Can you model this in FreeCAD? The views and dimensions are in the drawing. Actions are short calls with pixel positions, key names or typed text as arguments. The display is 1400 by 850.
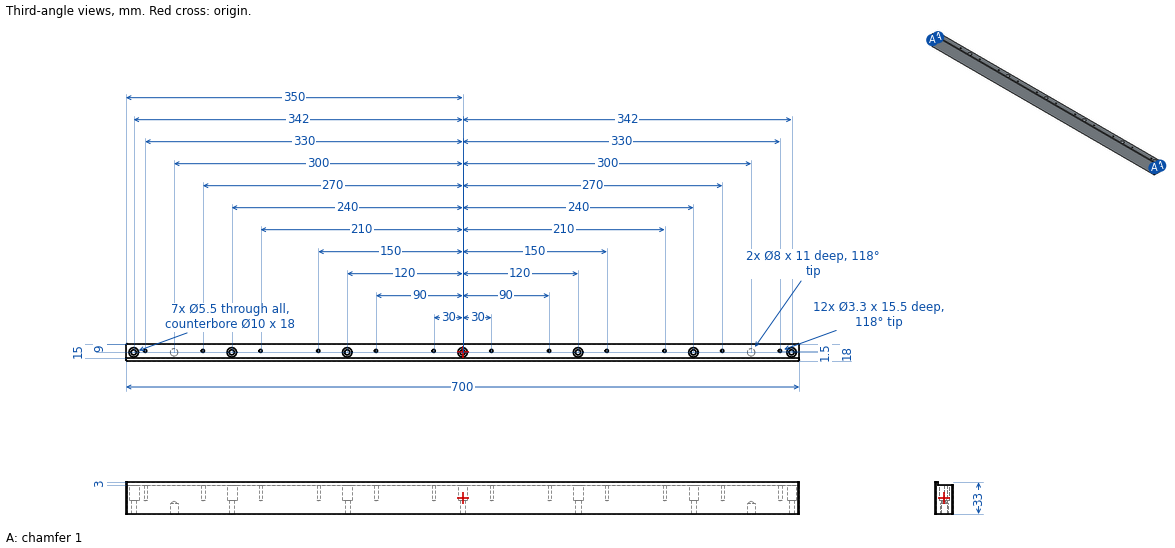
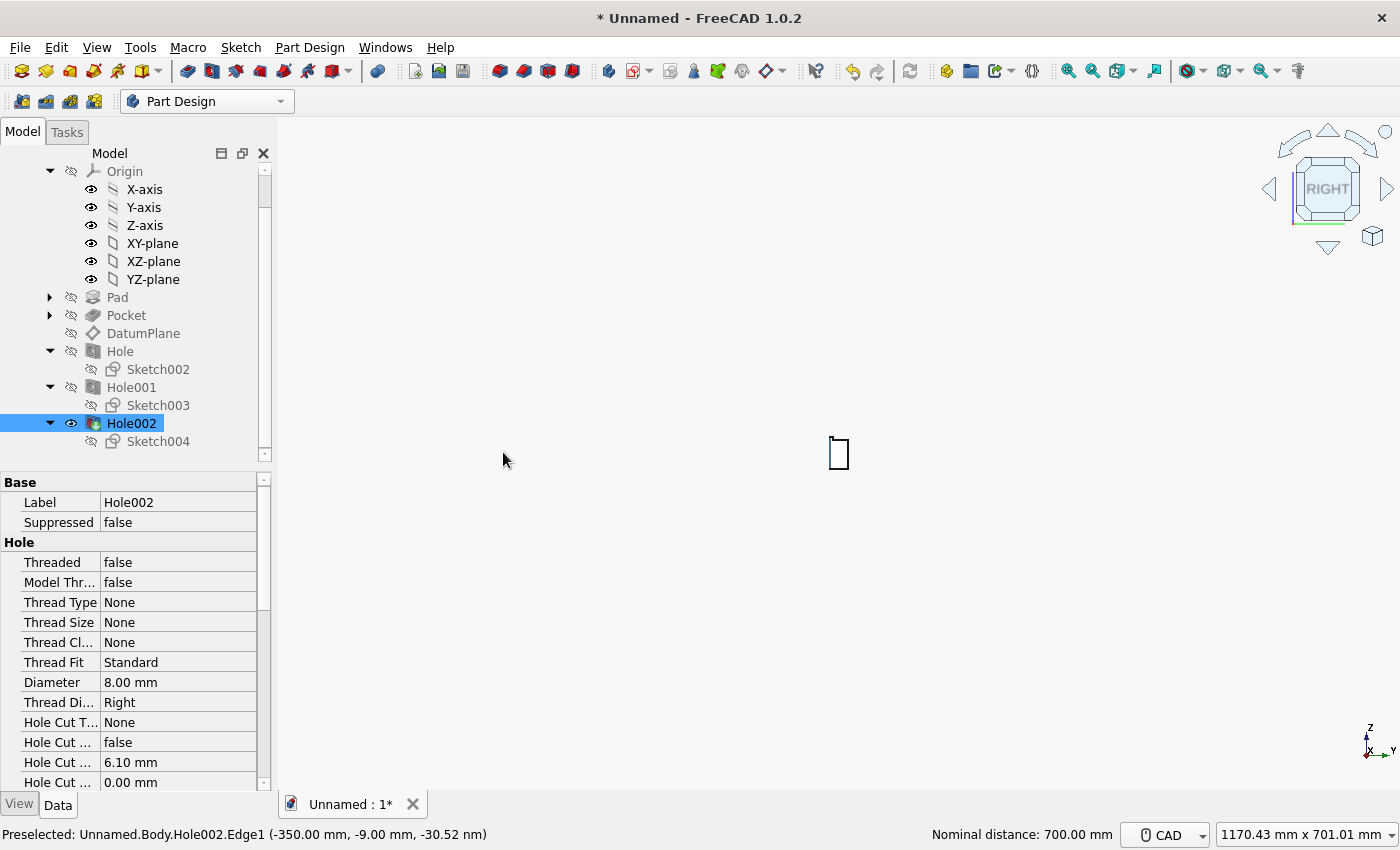
key(v)
key(f)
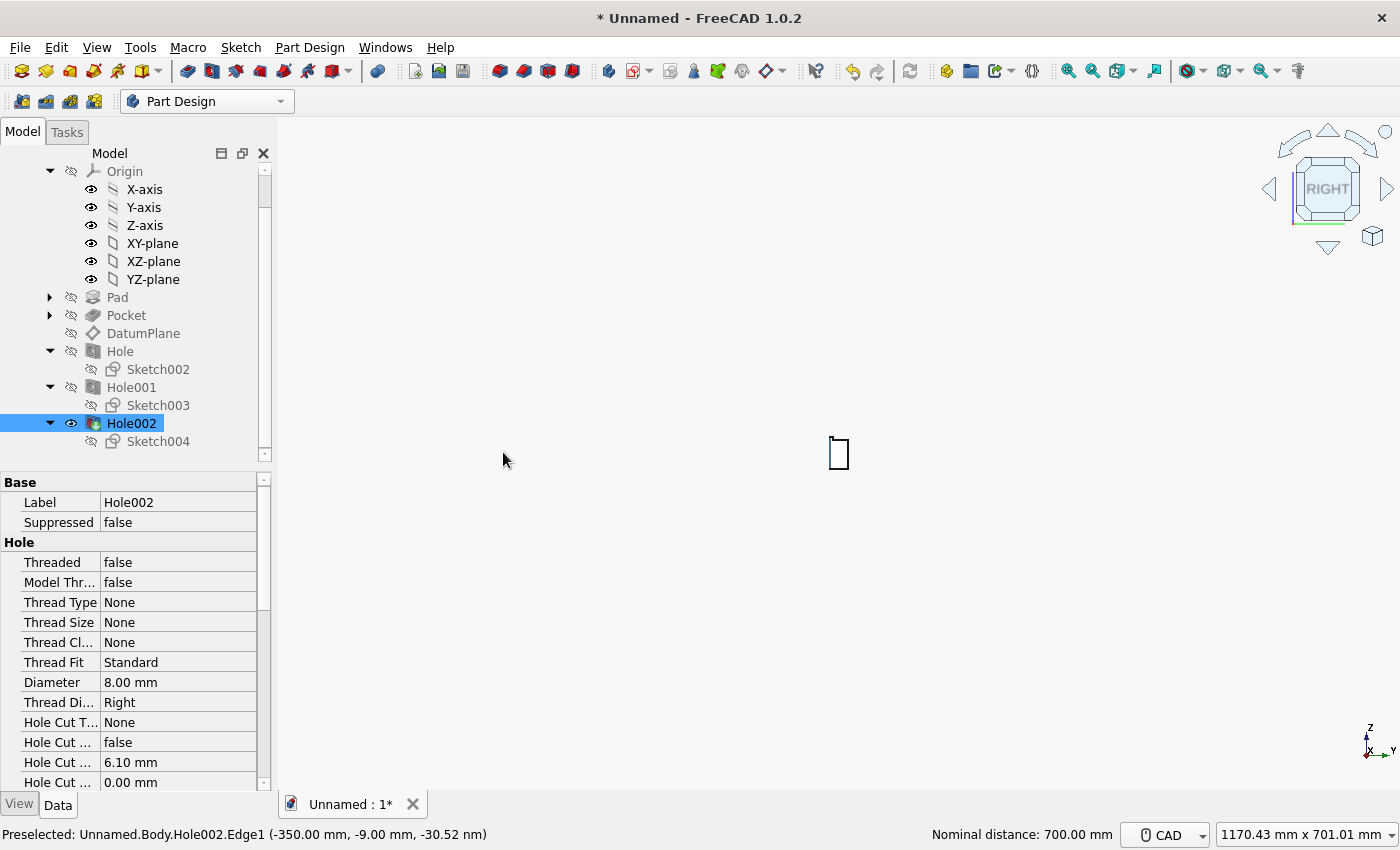
click(848, 453, ctrl)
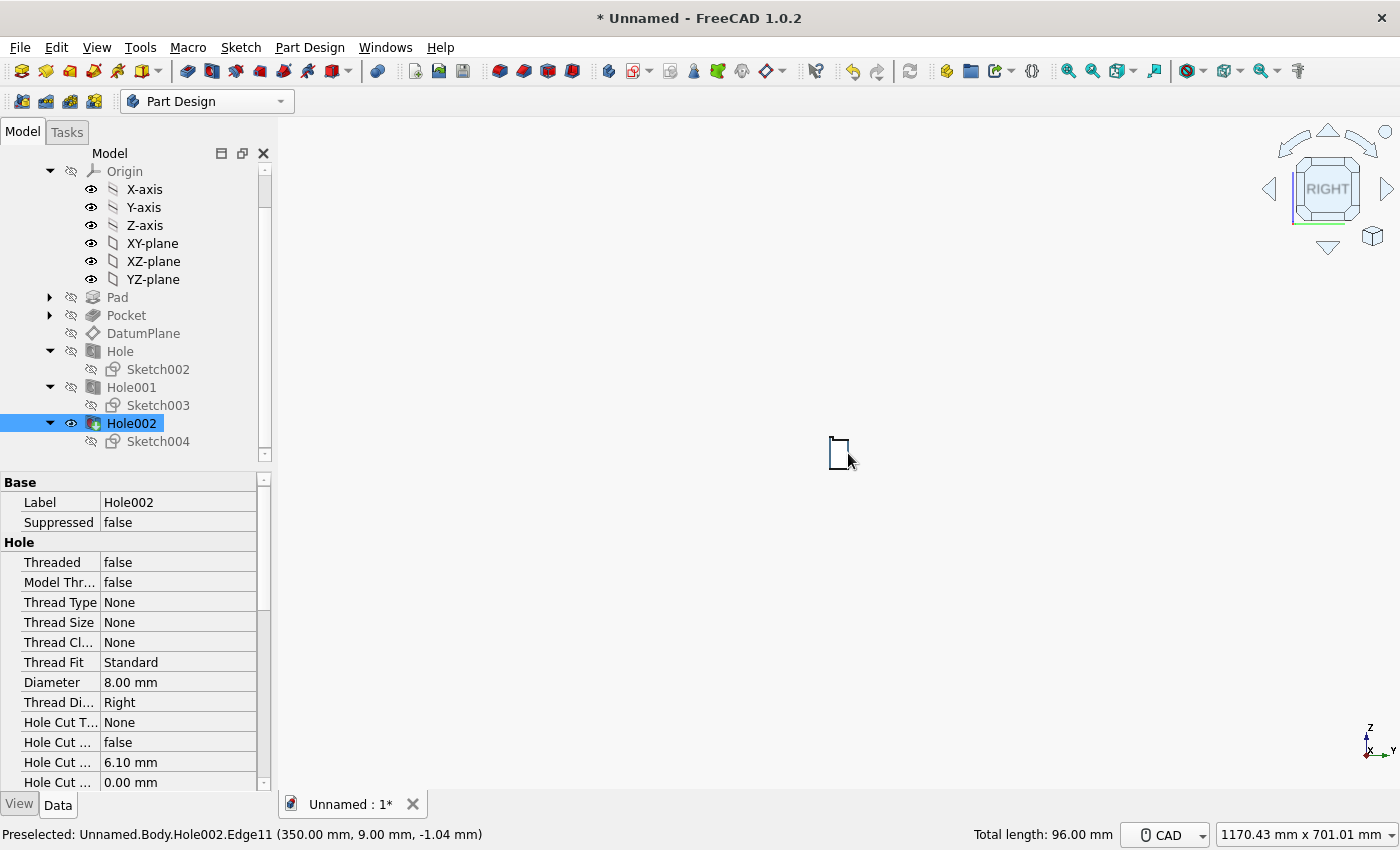
key(5)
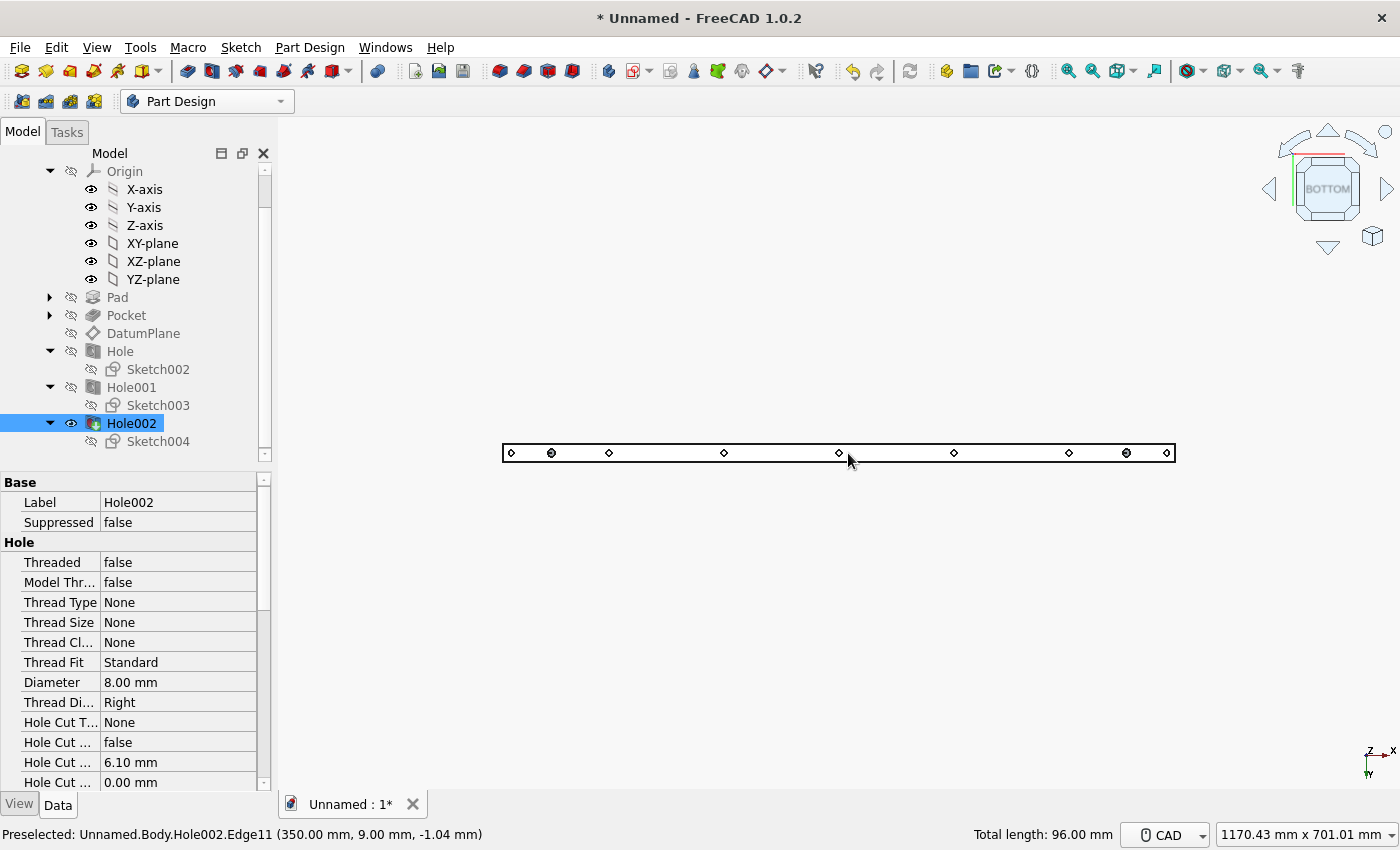
key(4)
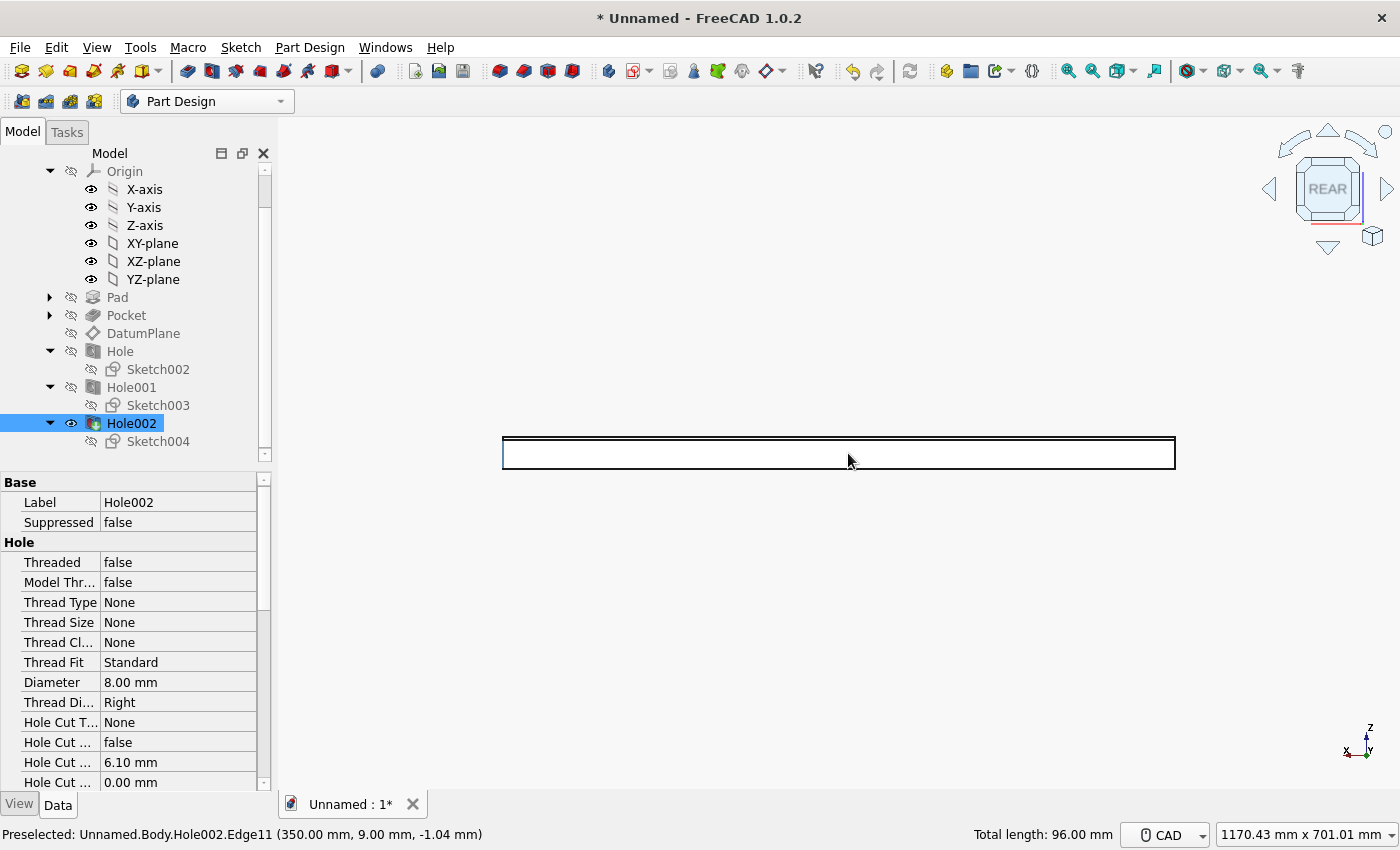
click(1175, 453, ctrl)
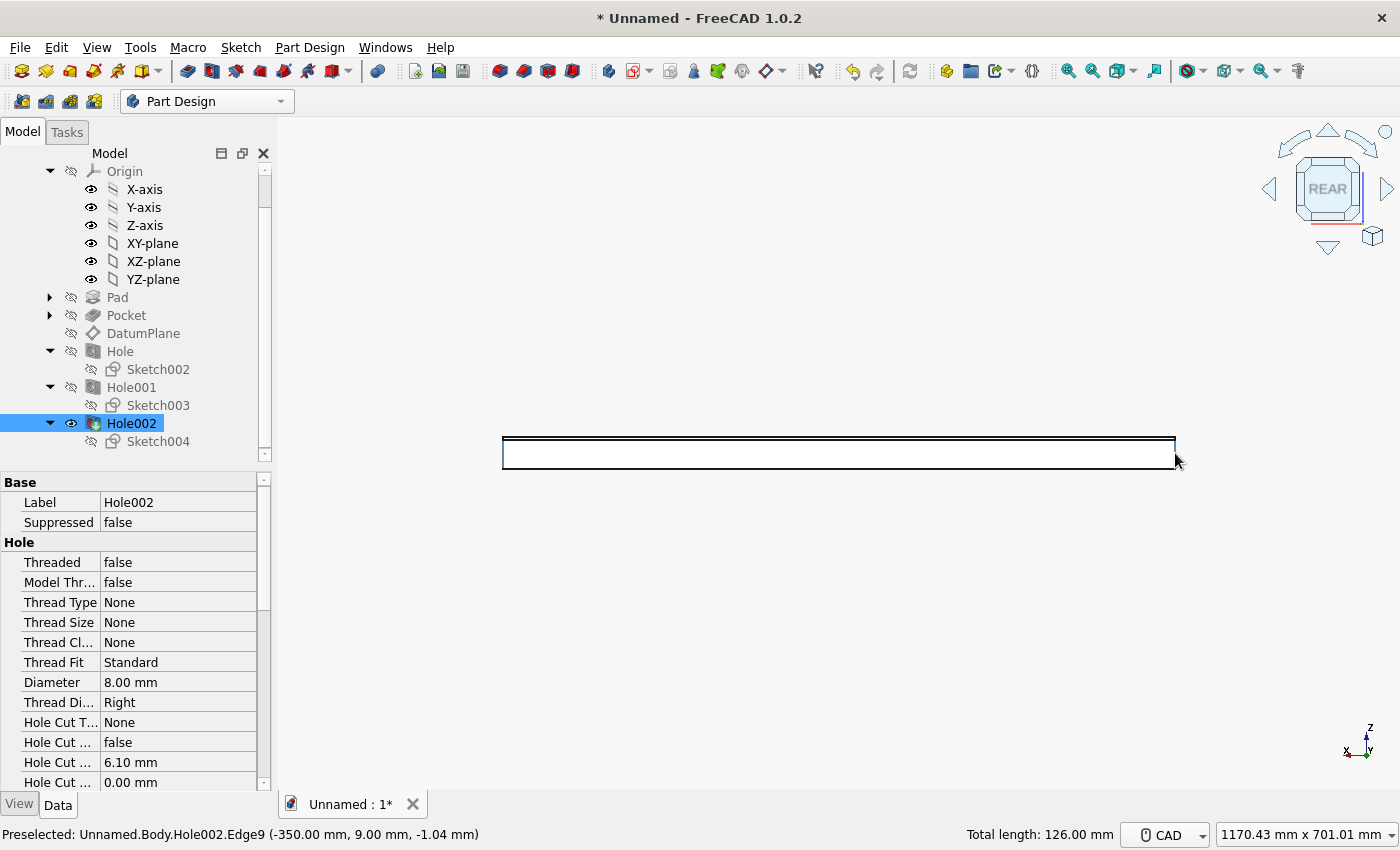
click(524, 72)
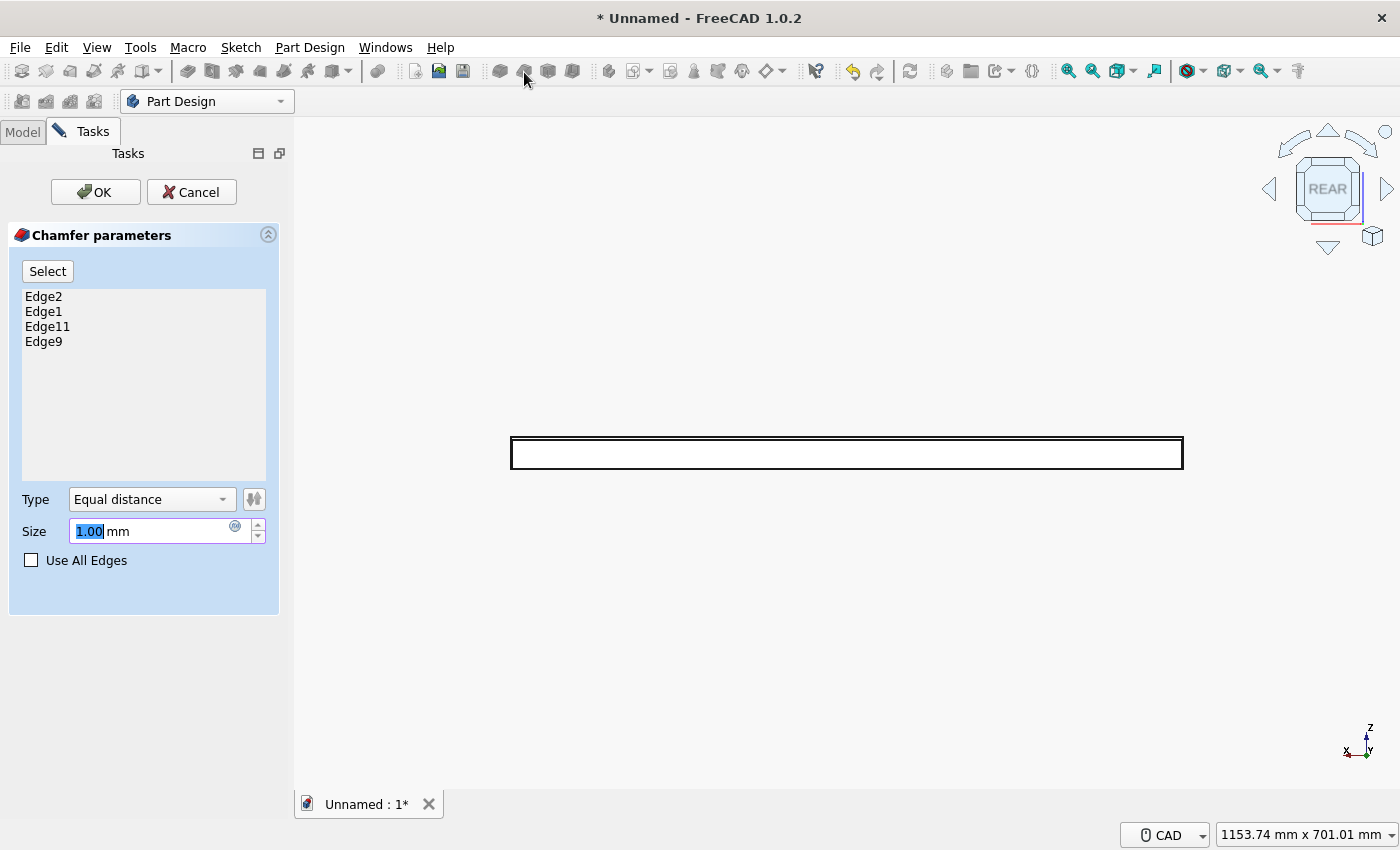
text(1)
key(Tab)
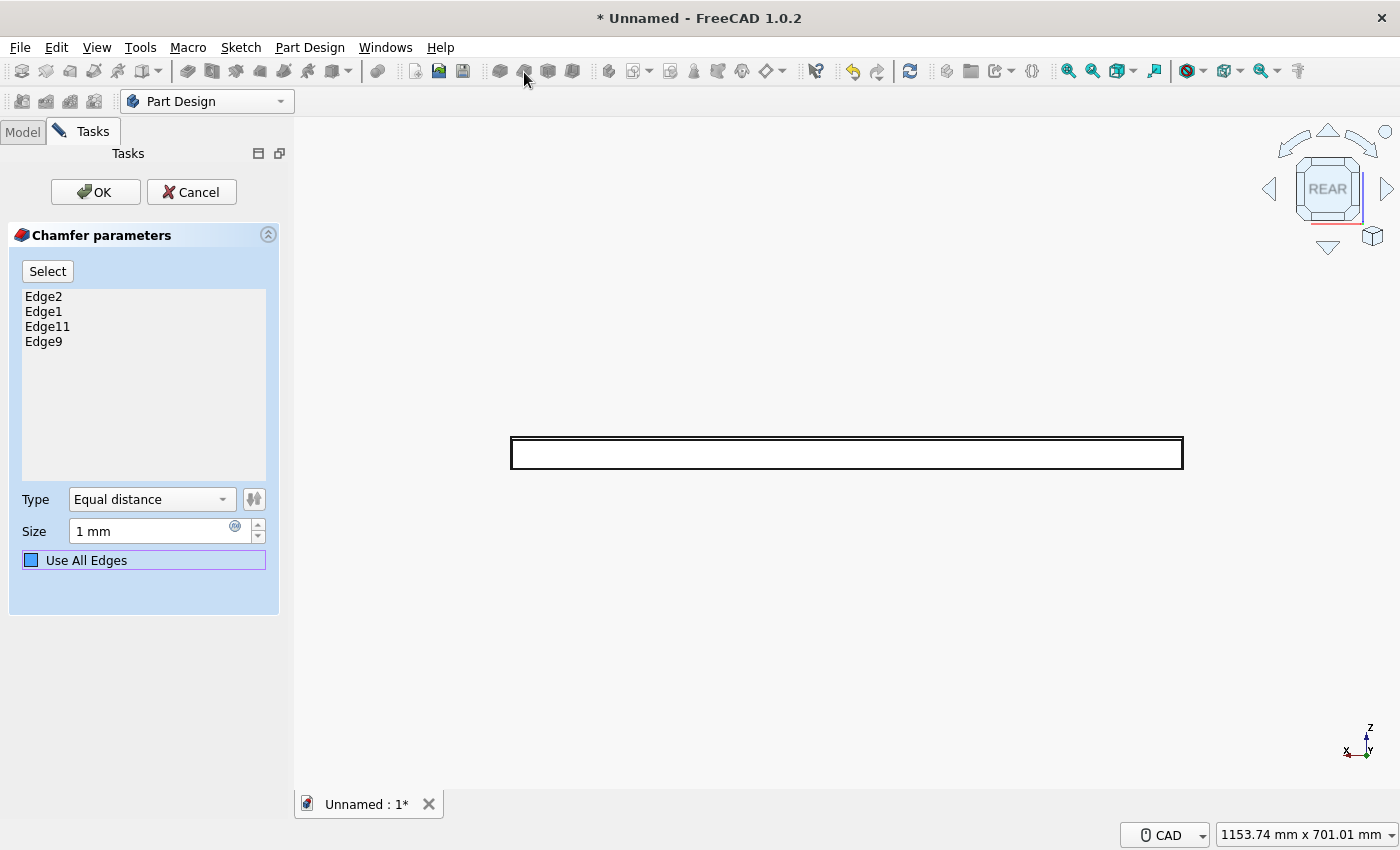
click(96, 192)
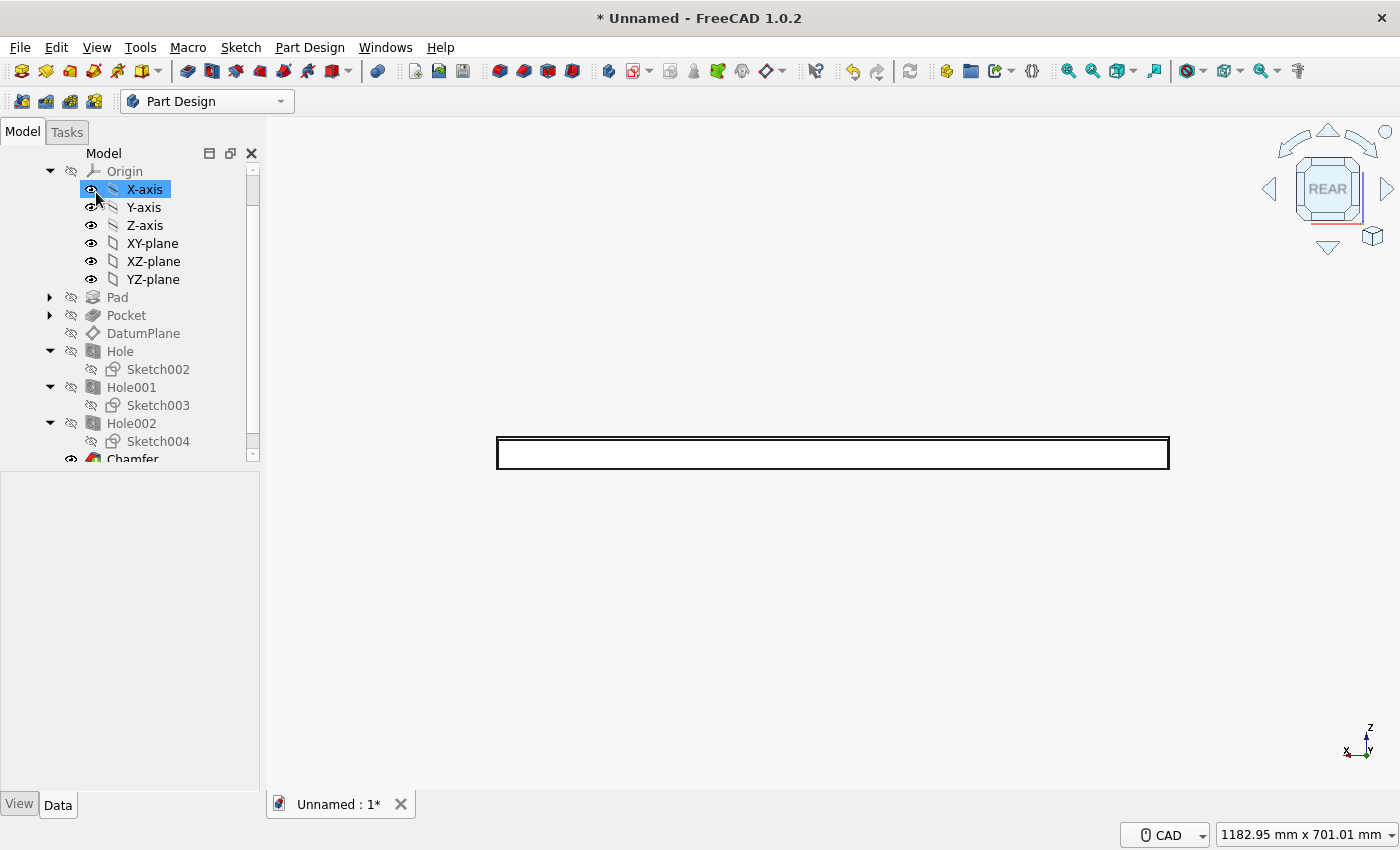
key(0)